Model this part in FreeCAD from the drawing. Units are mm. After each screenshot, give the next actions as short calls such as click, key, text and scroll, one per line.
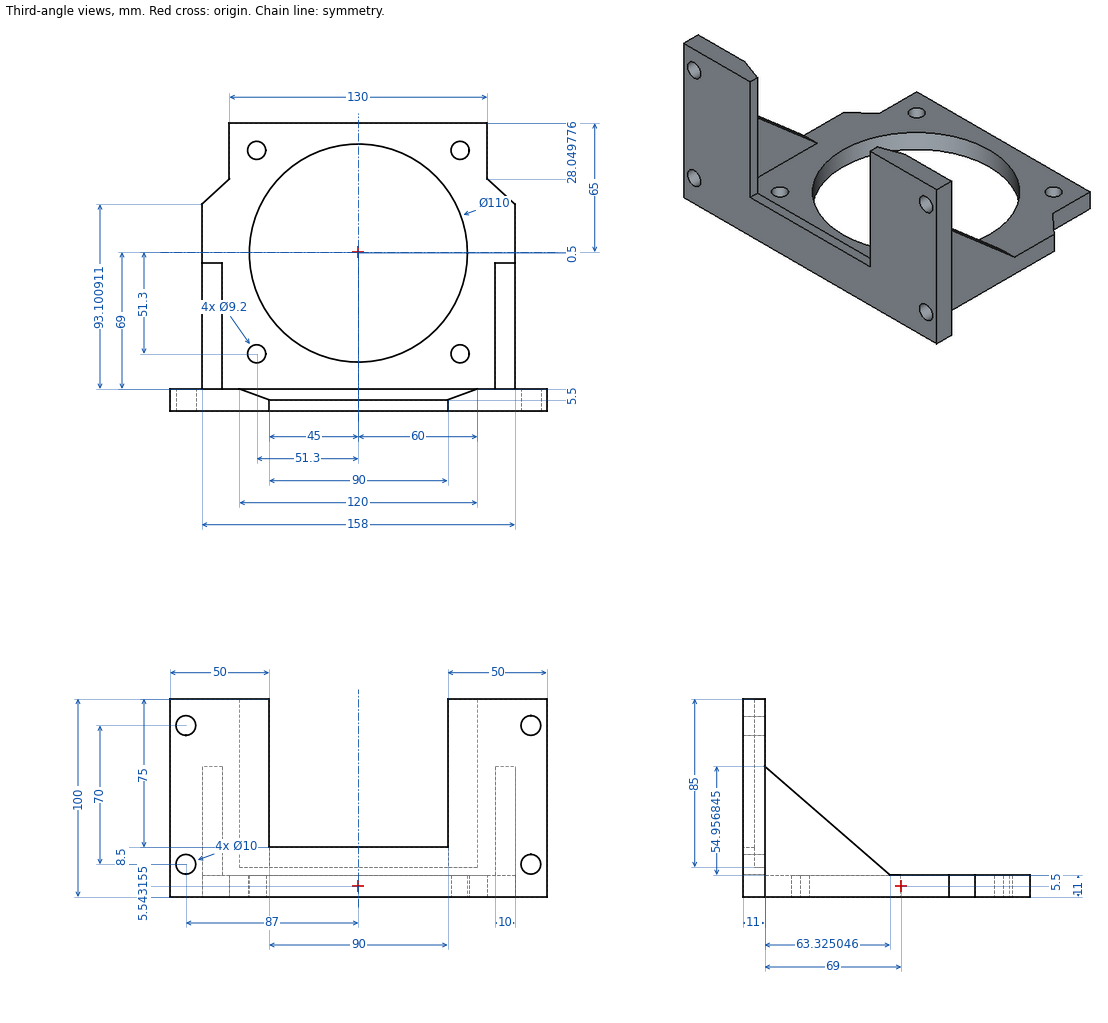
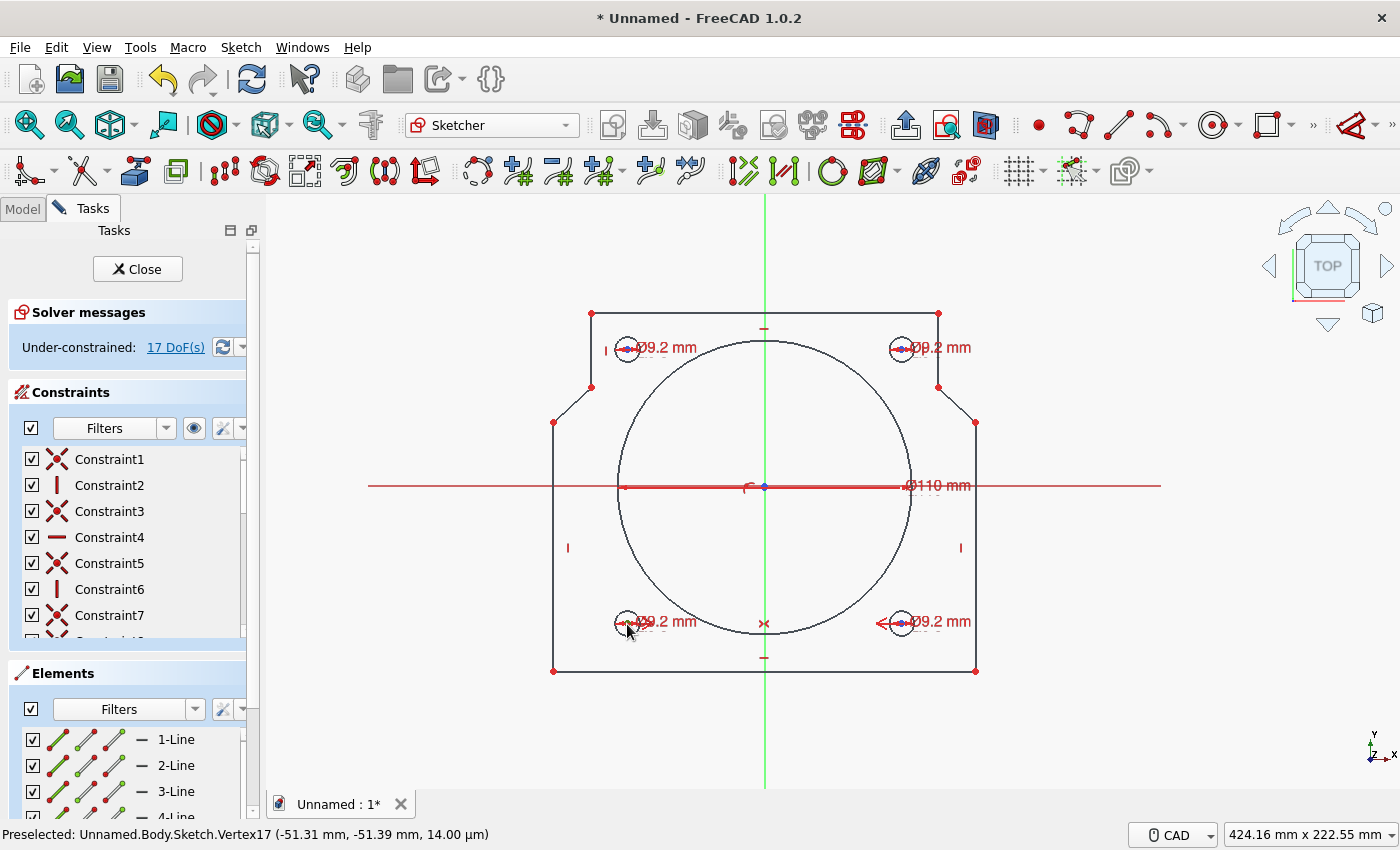
click(628, 350)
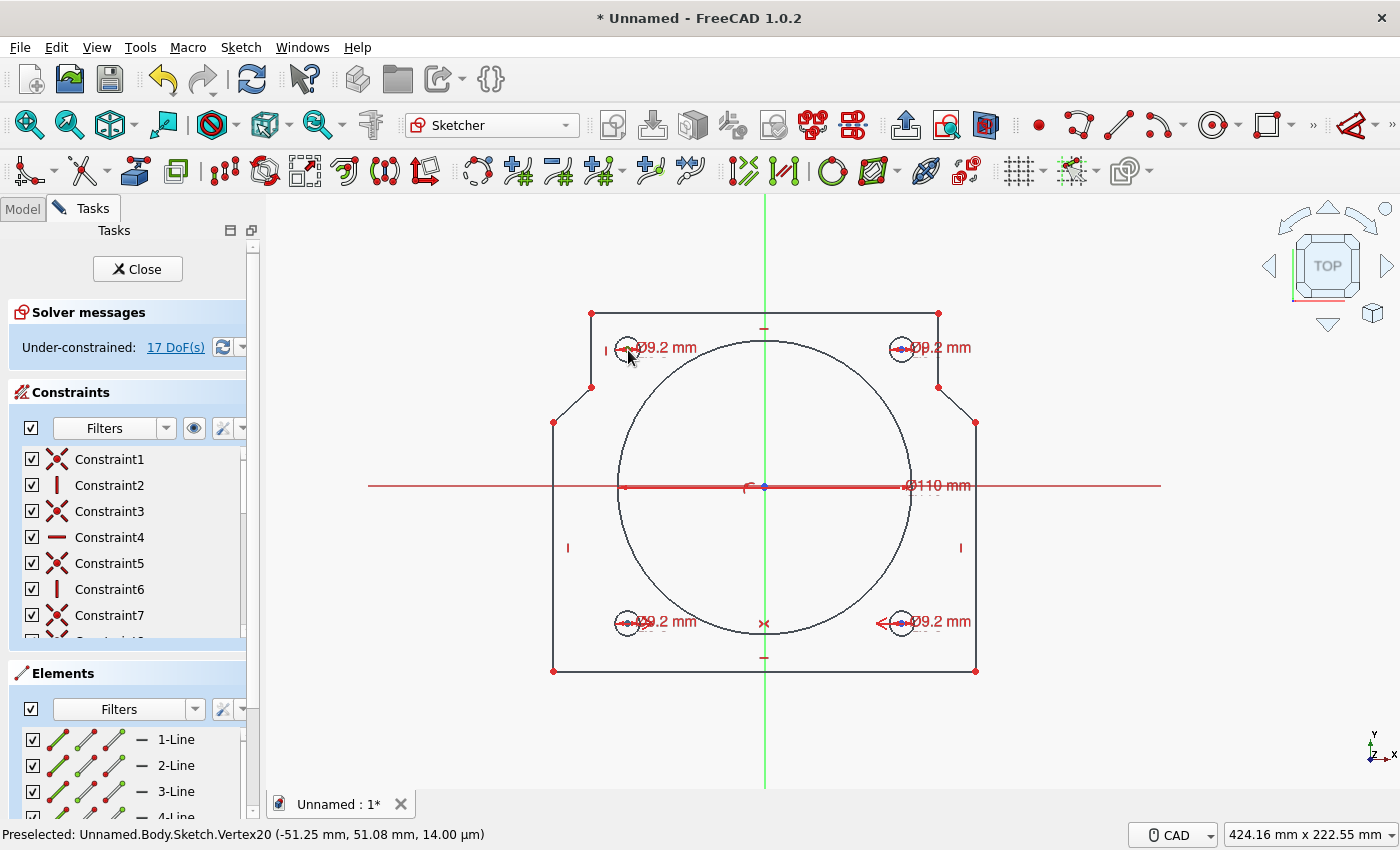
click(428, 486)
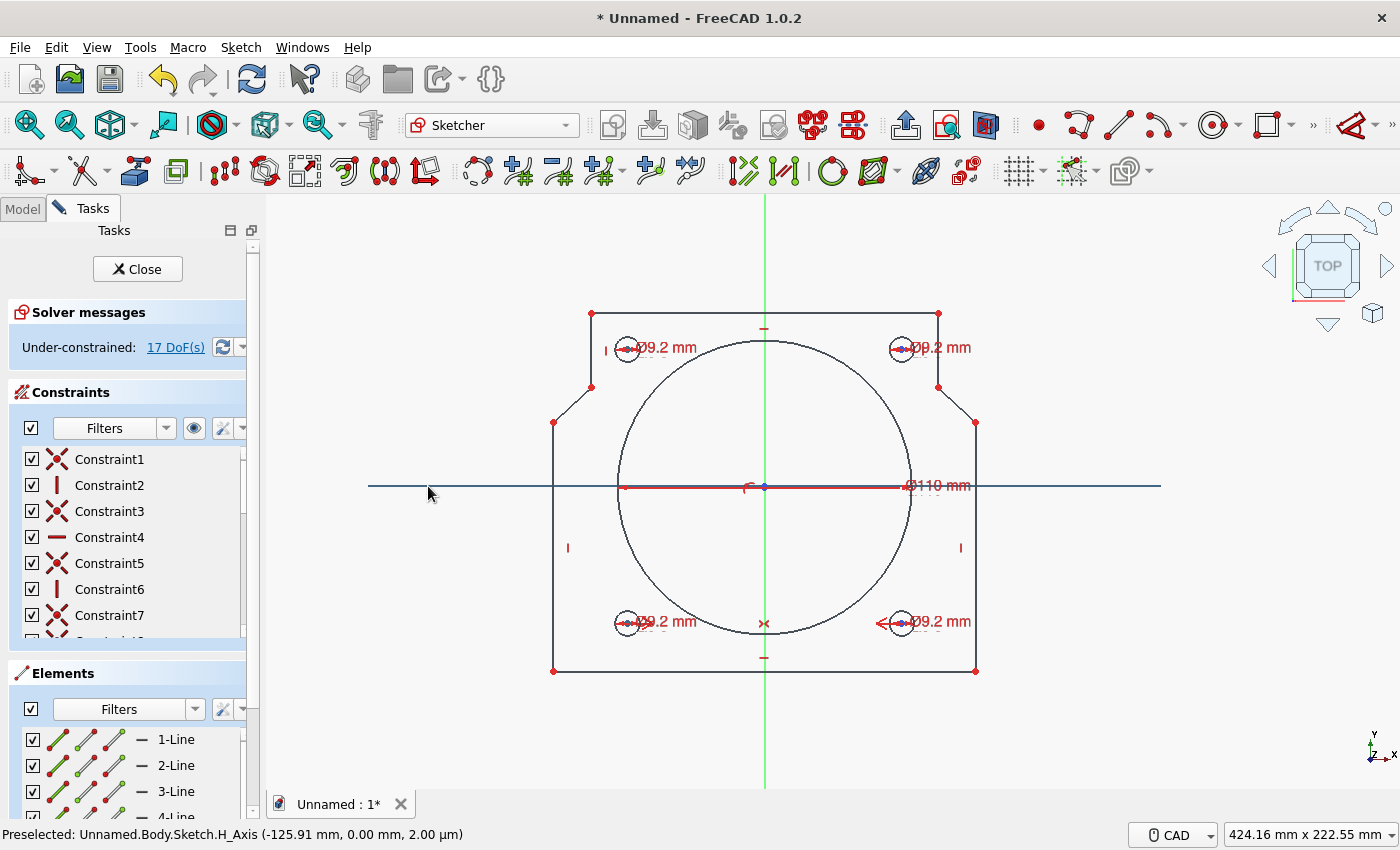
key(s)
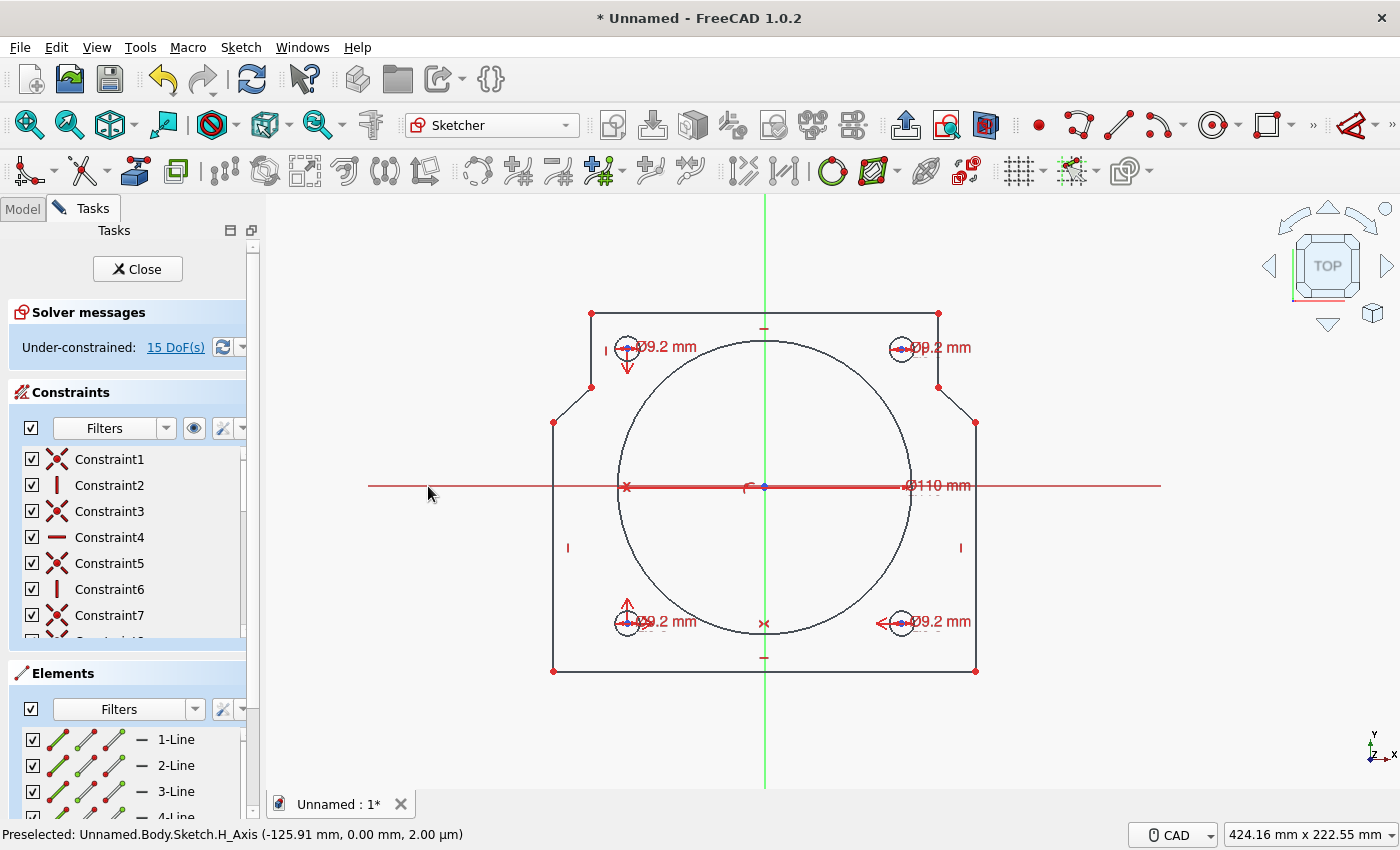
click(902, 624)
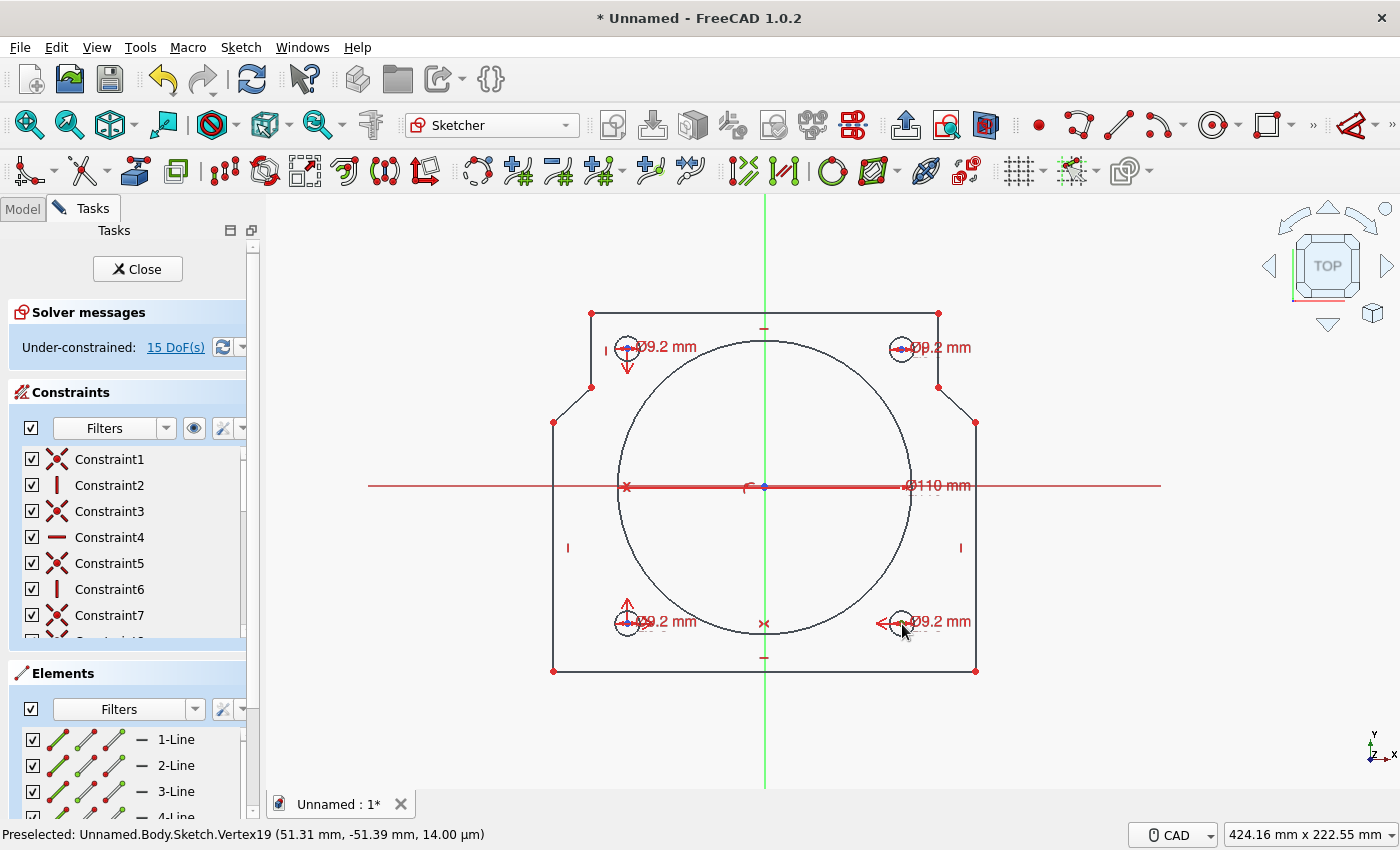
click(902, 350)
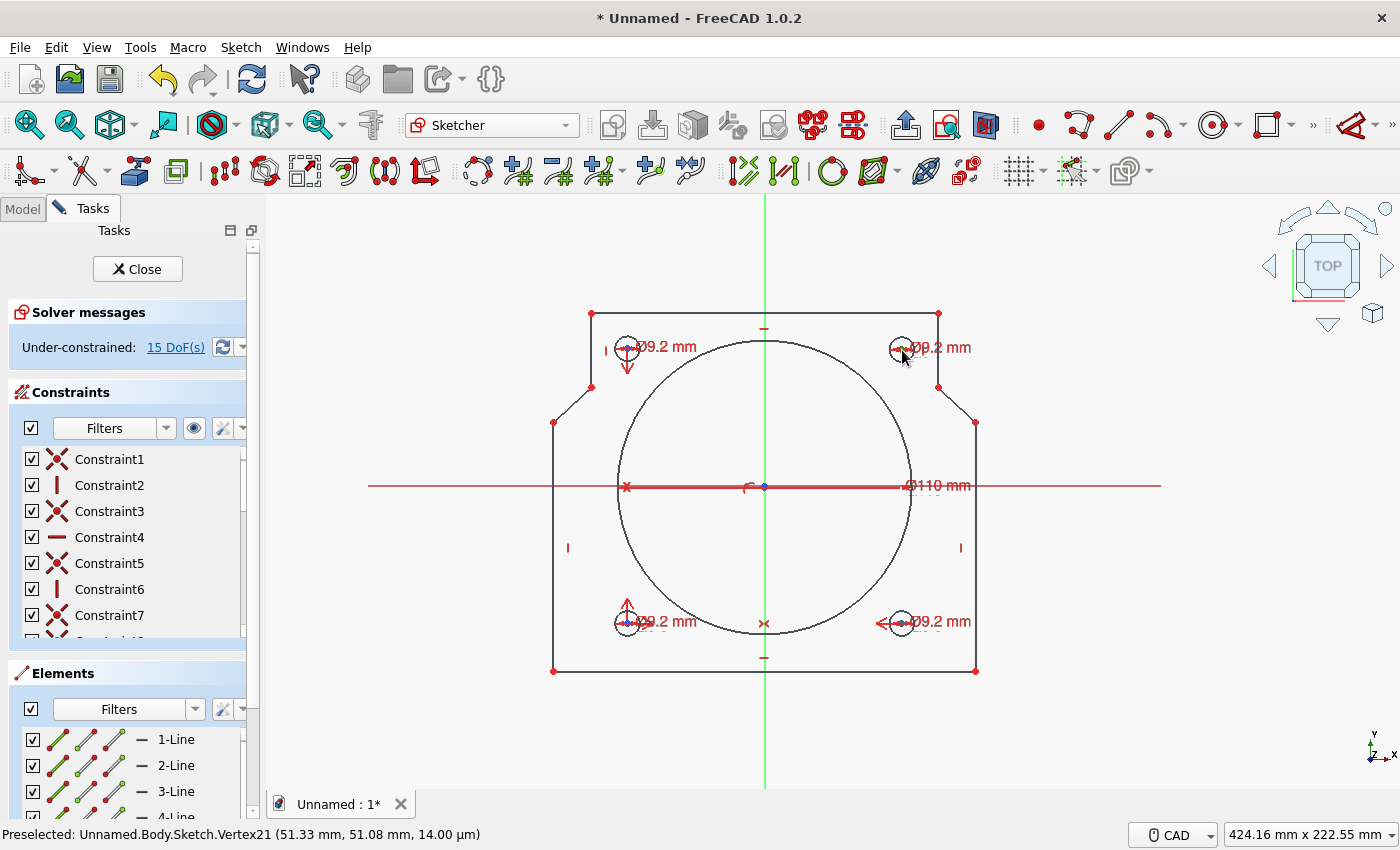
click(428, 486)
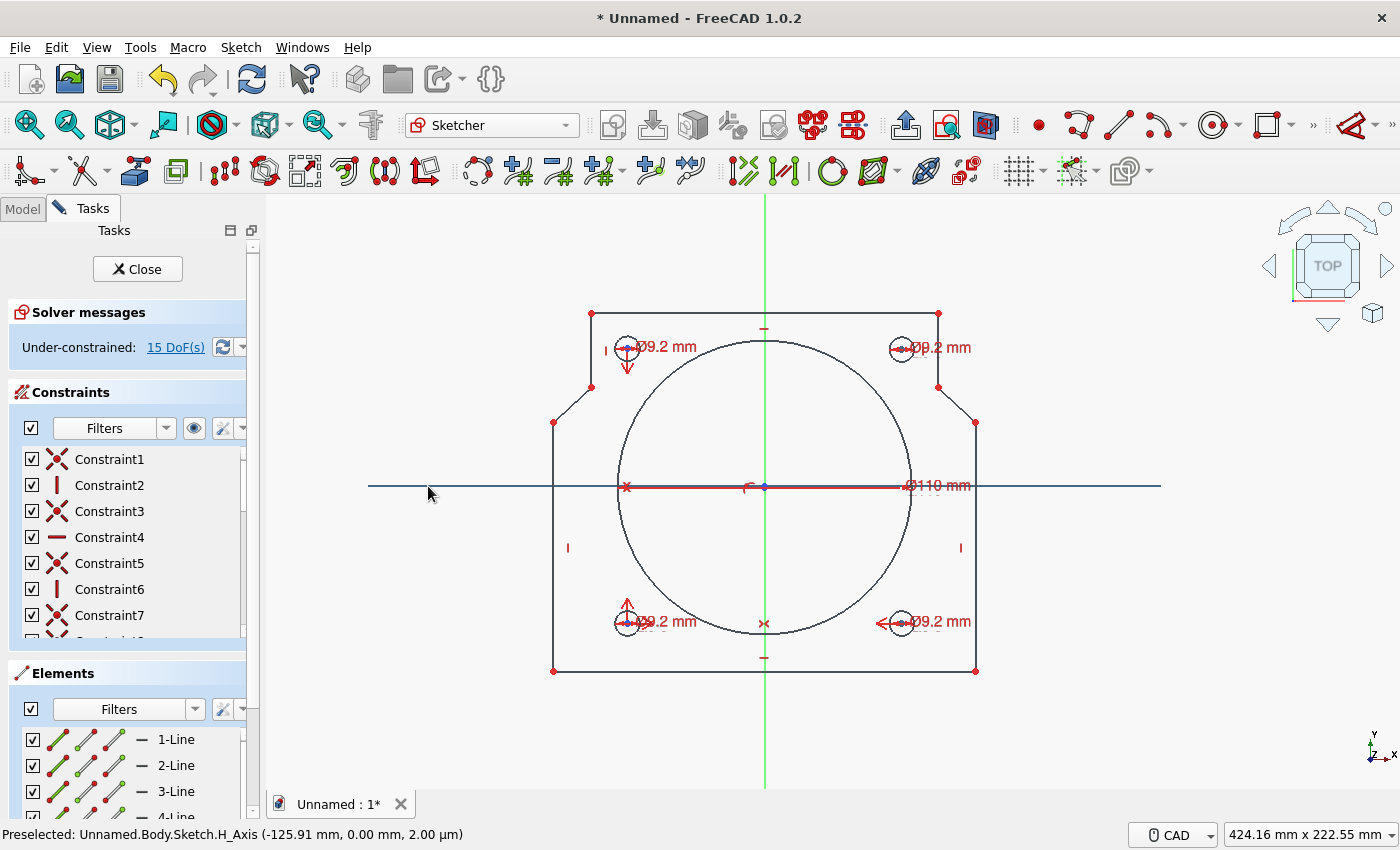
key(s)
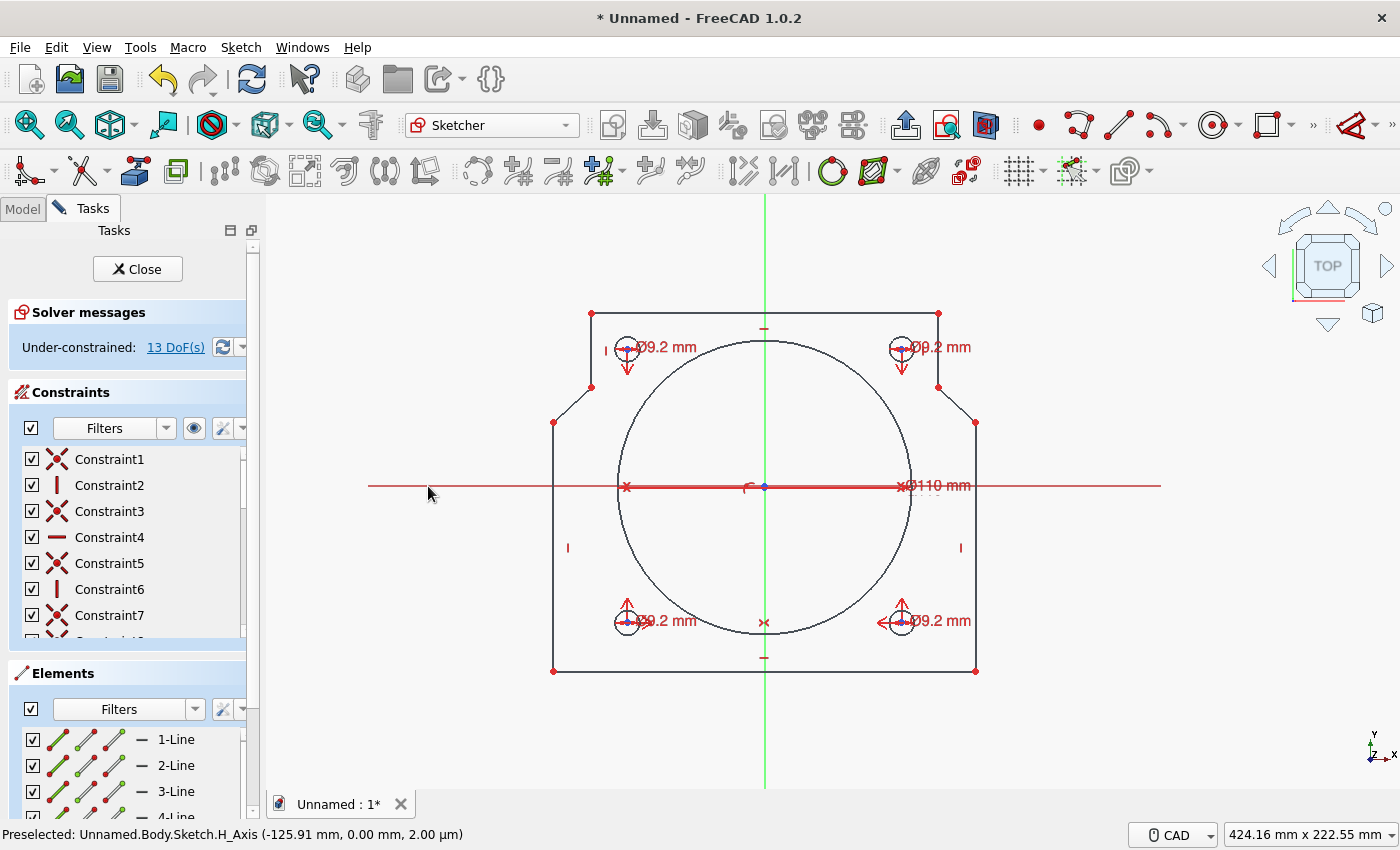
click(553, 423)